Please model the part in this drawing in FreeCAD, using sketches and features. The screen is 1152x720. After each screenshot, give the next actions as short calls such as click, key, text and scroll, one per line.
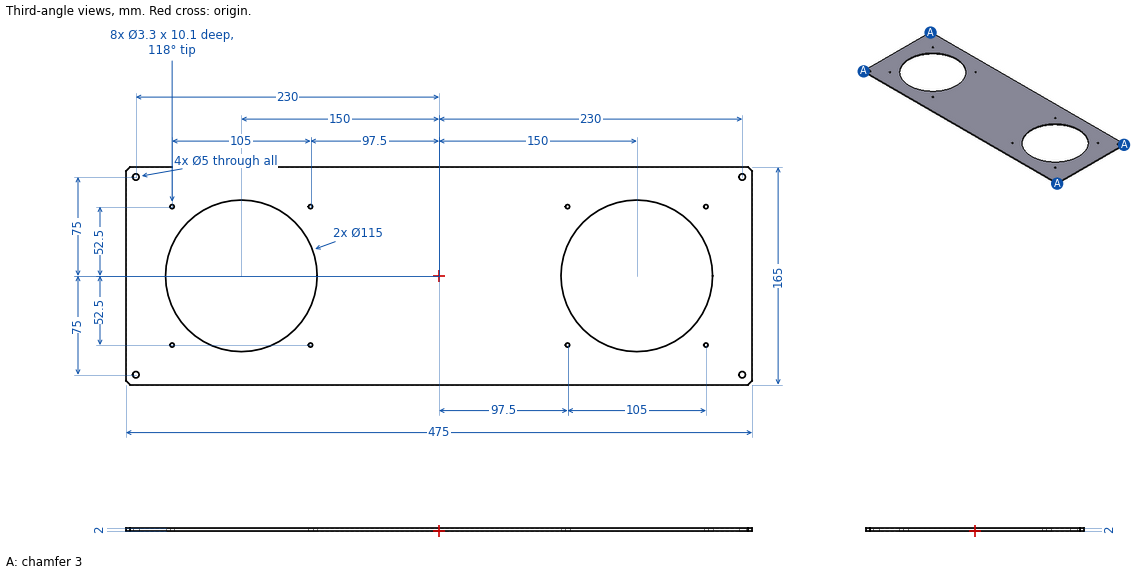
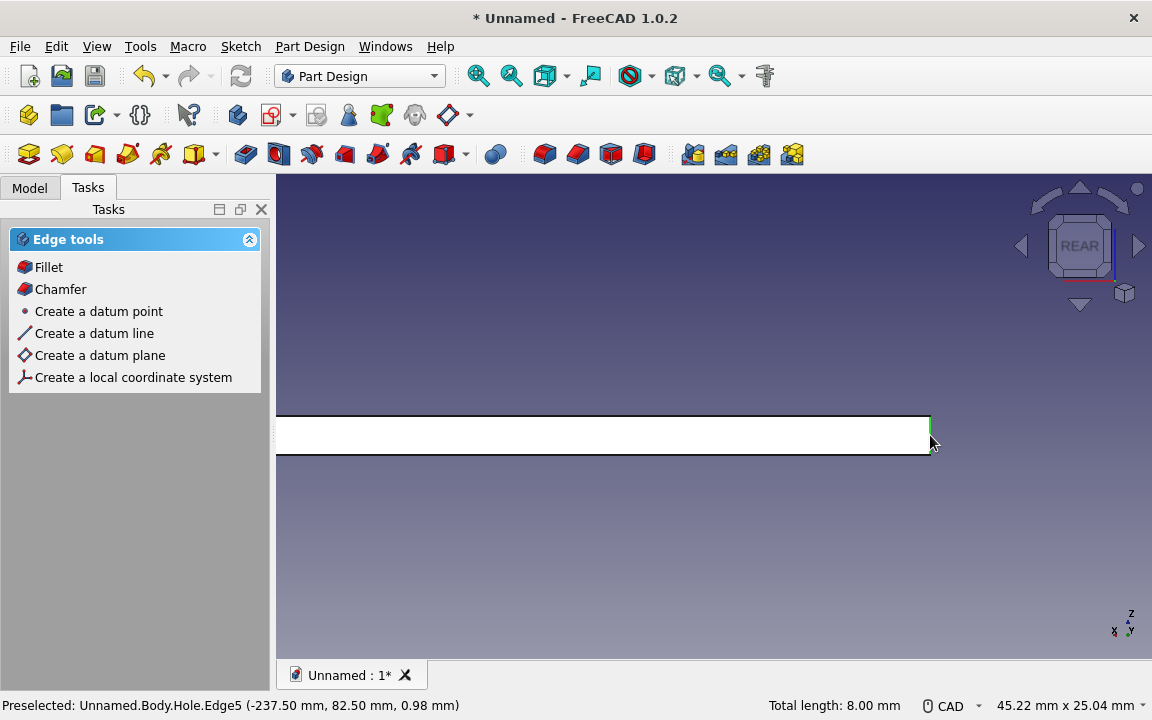
click(578, 154)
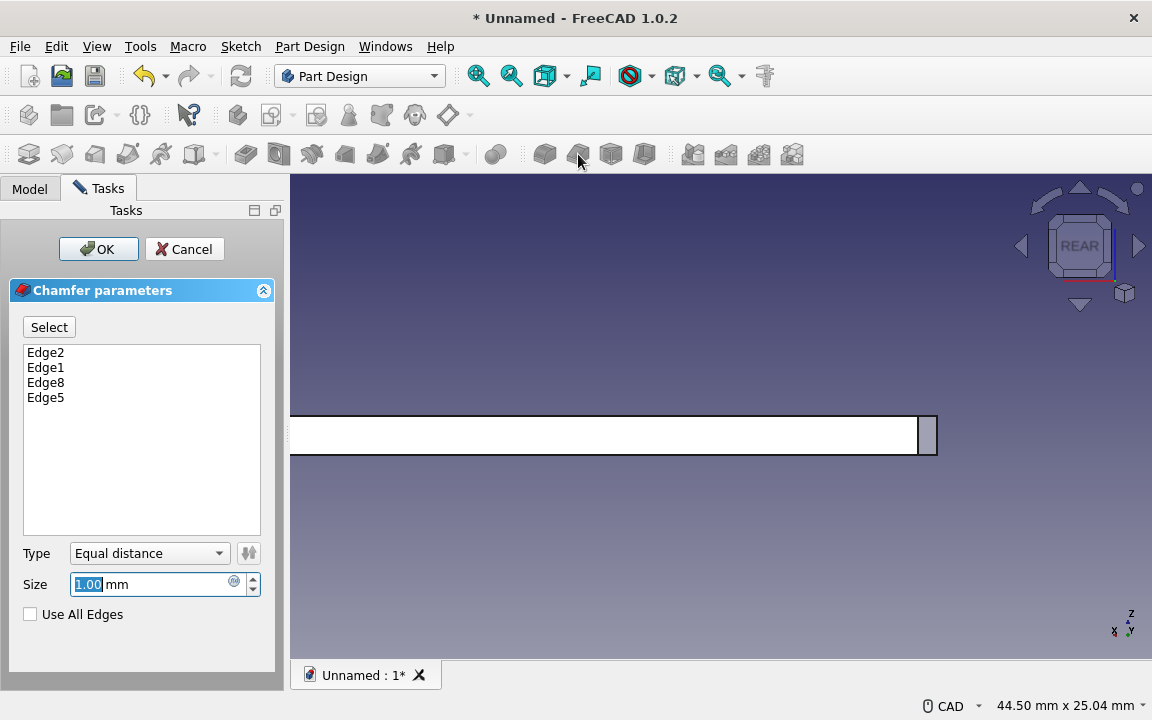
text(3)
key(Tab)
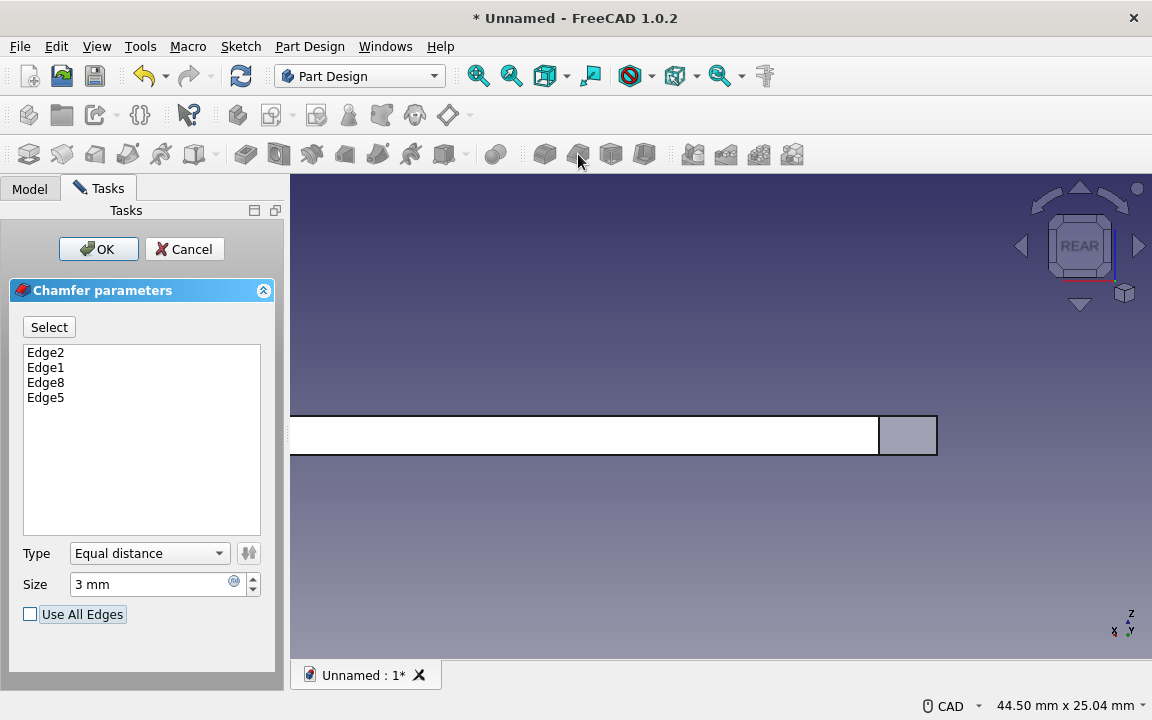
click(99, 249)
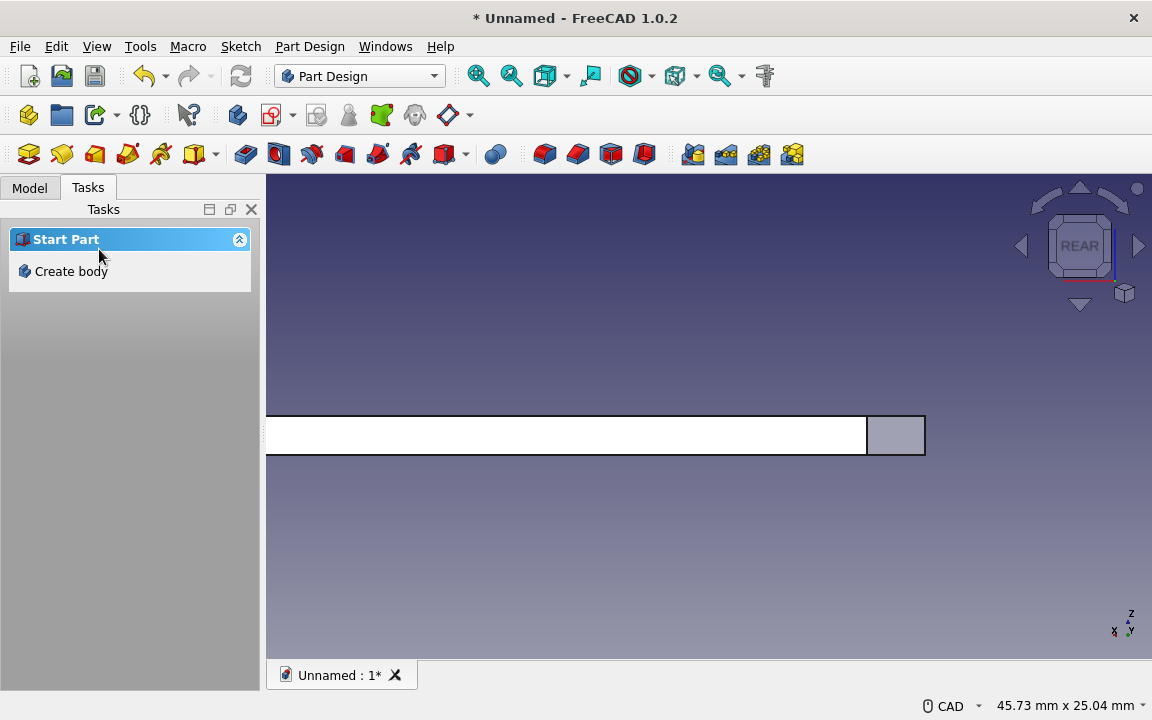
key(v)
key(f)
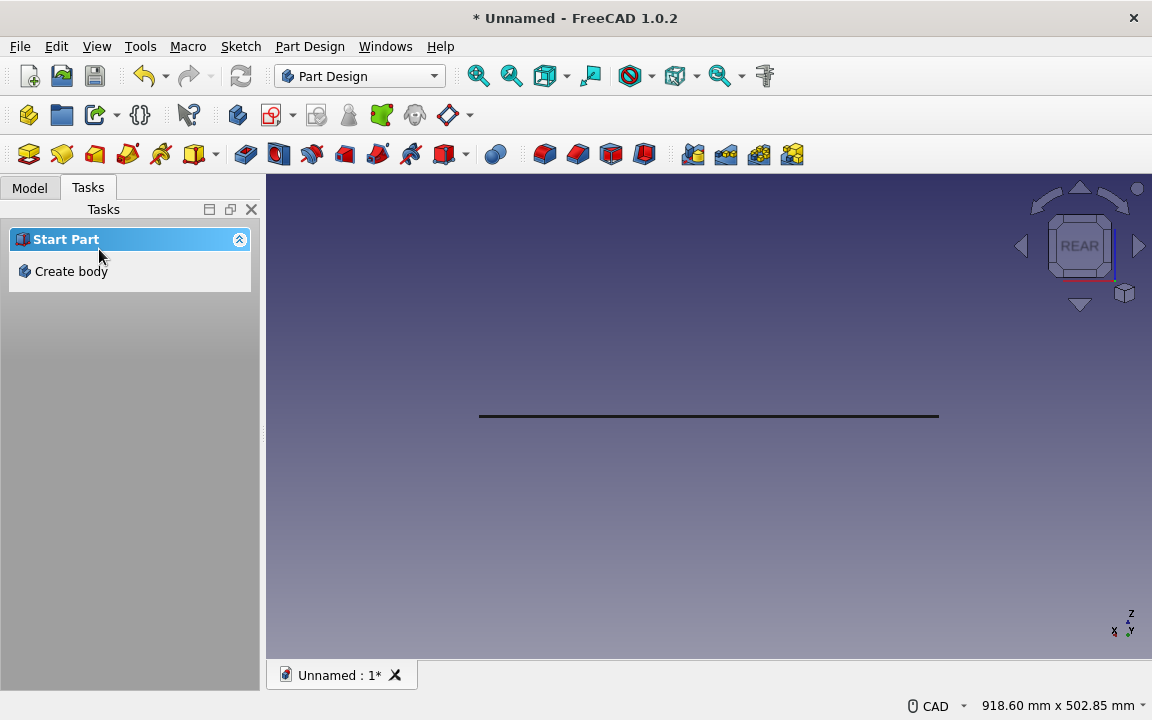
key(0)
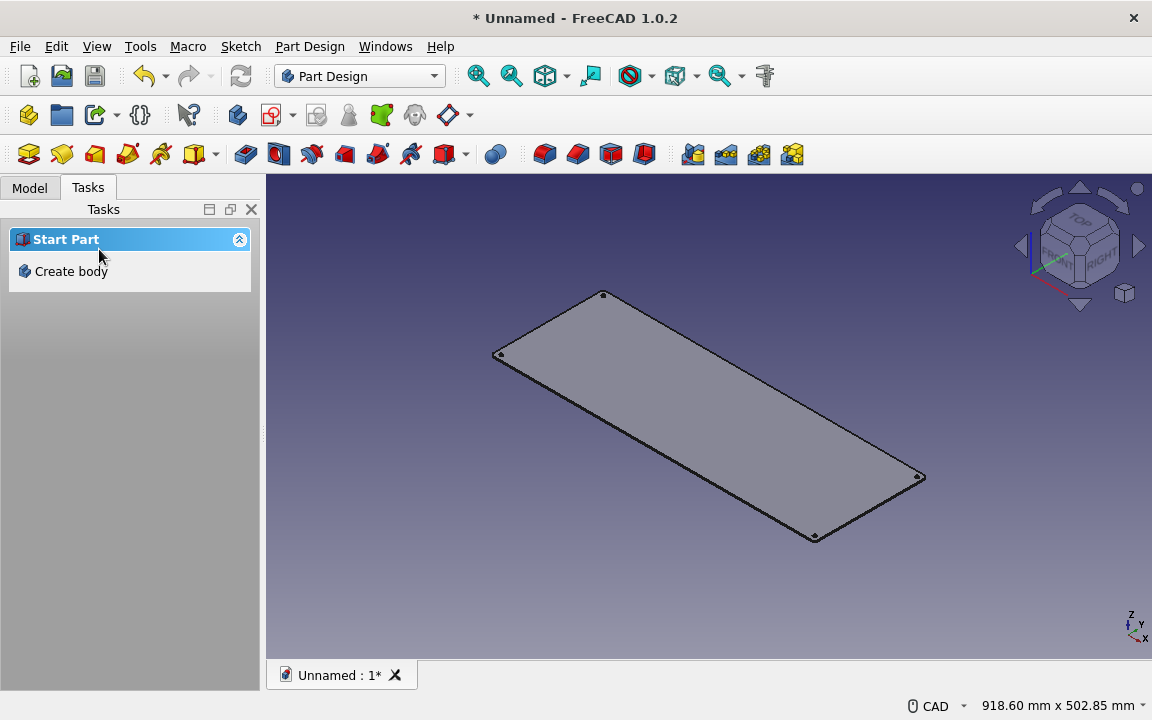
click(802, 468)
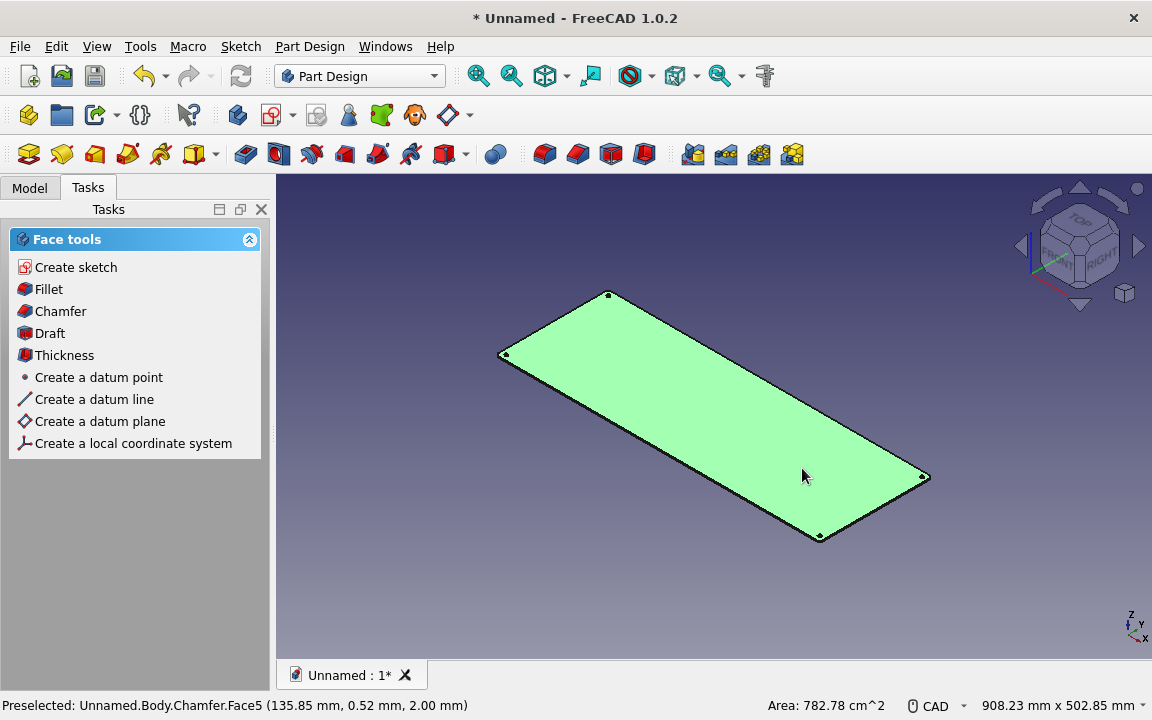
click(270, 116)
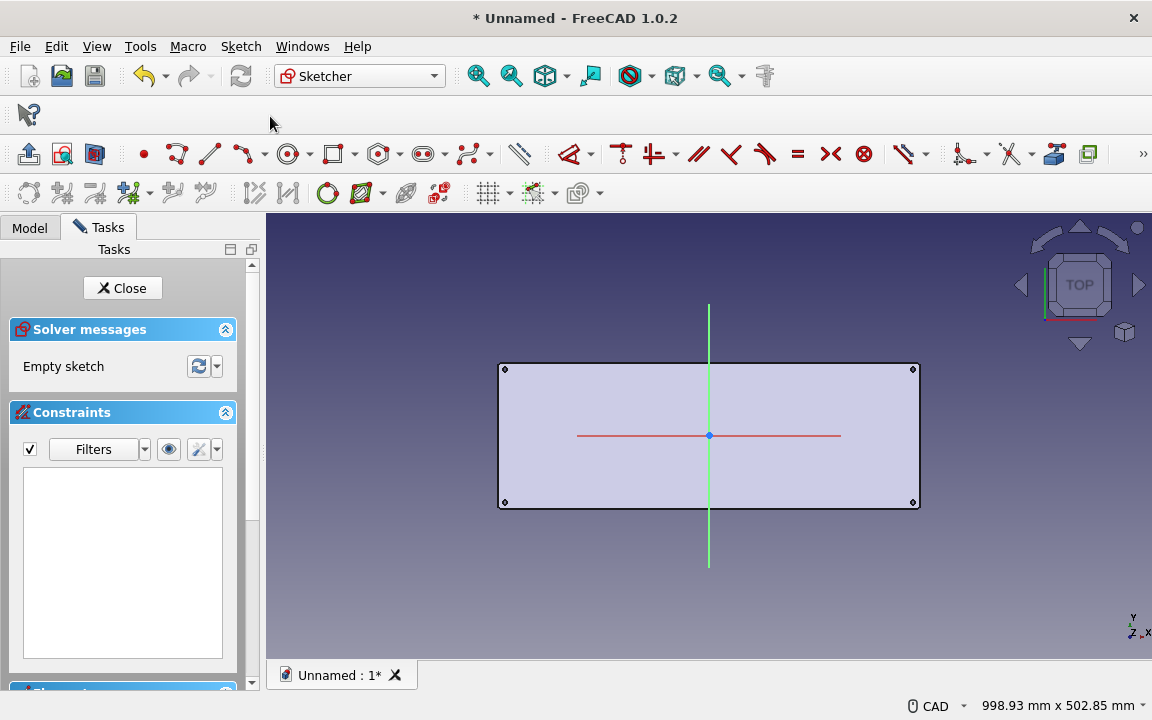
click(288, 154)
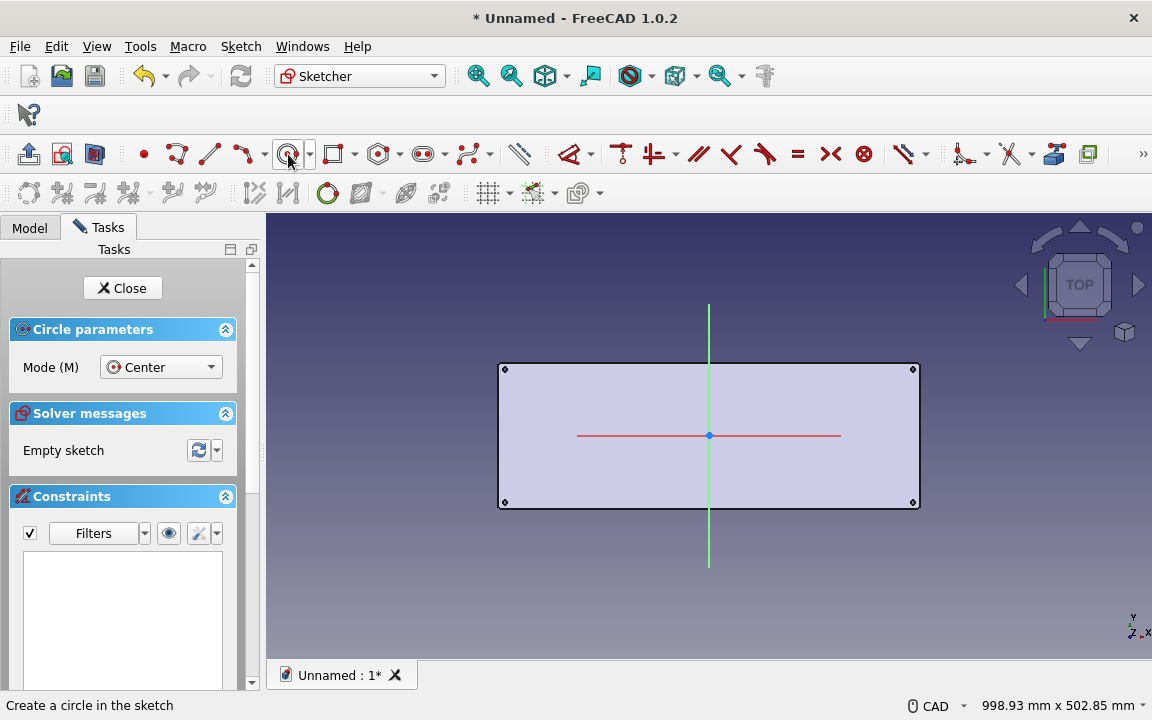
click(576, 436)
move(612, 400)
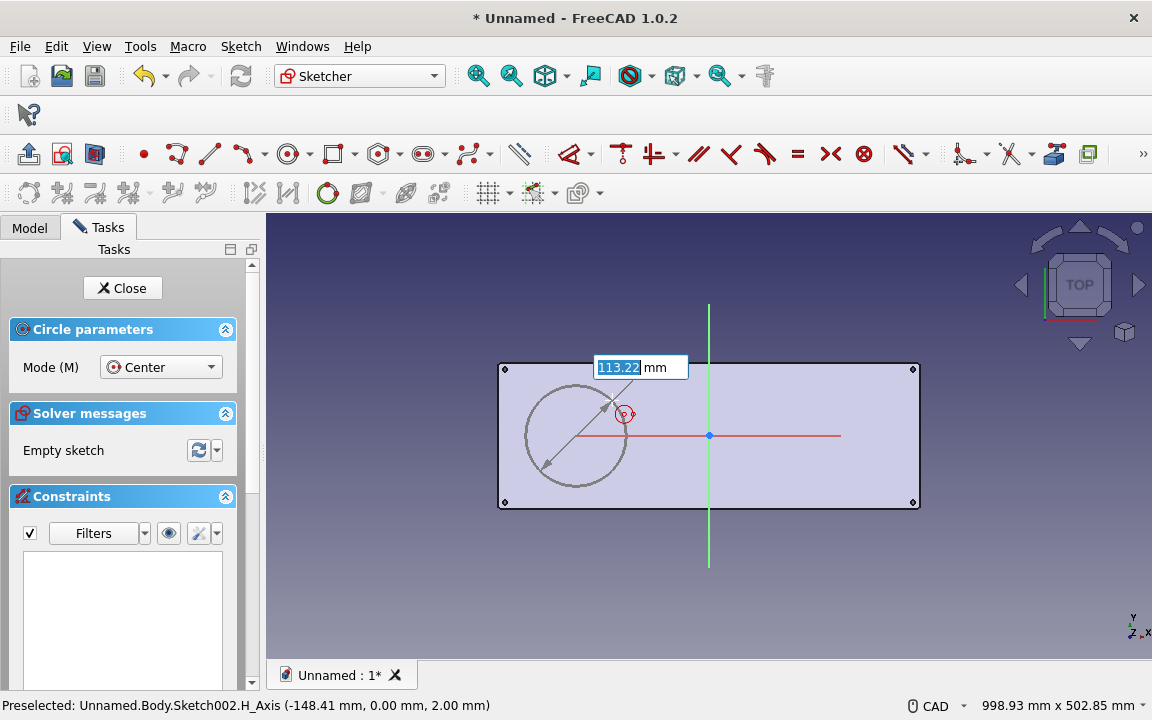
text(115)
key(Return)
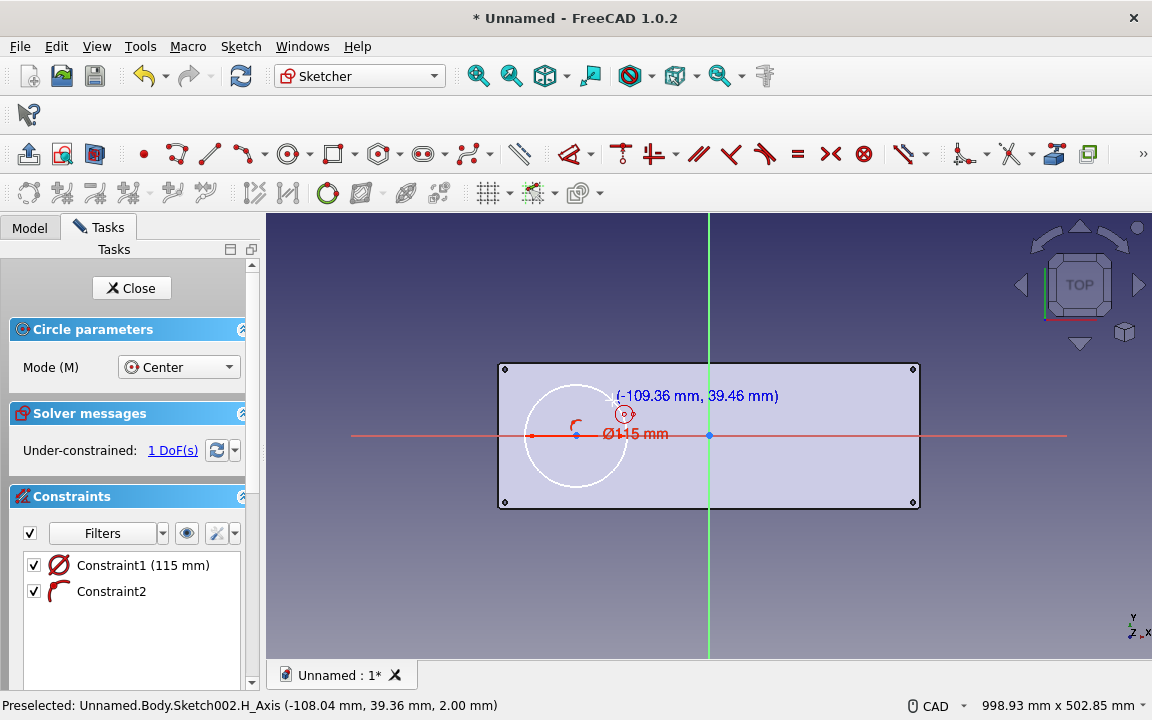
click(842, 436)
move(878, 400)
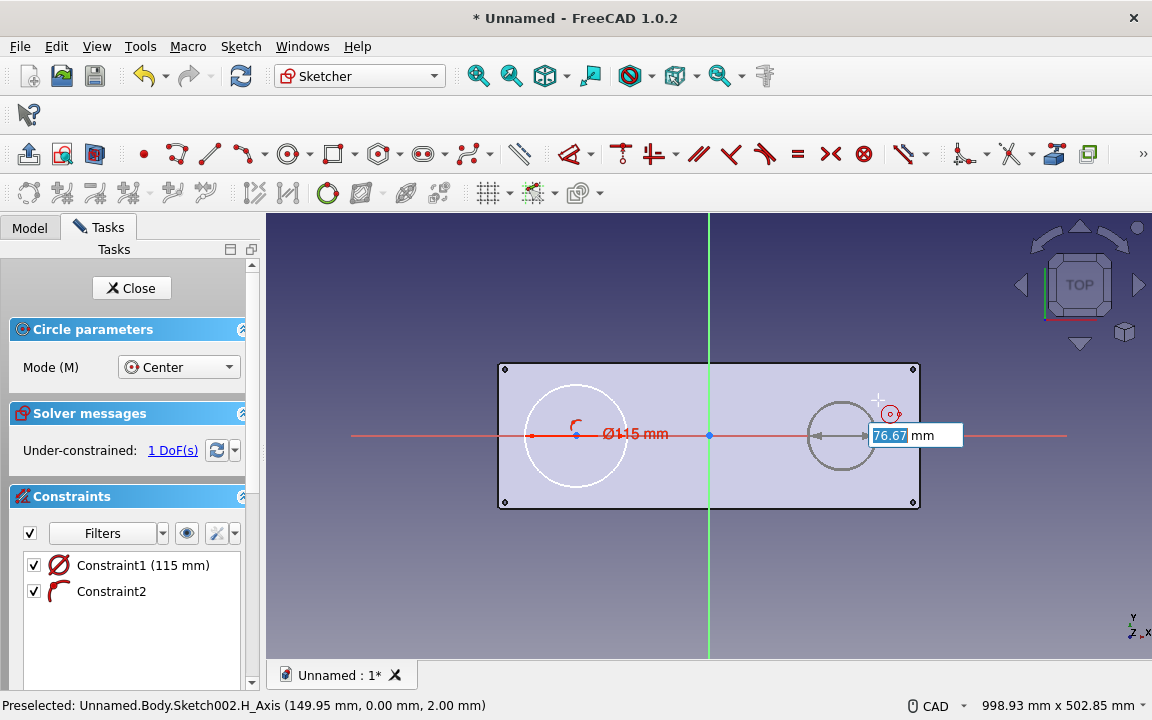
text(115)
key(Return)
key(Escape)